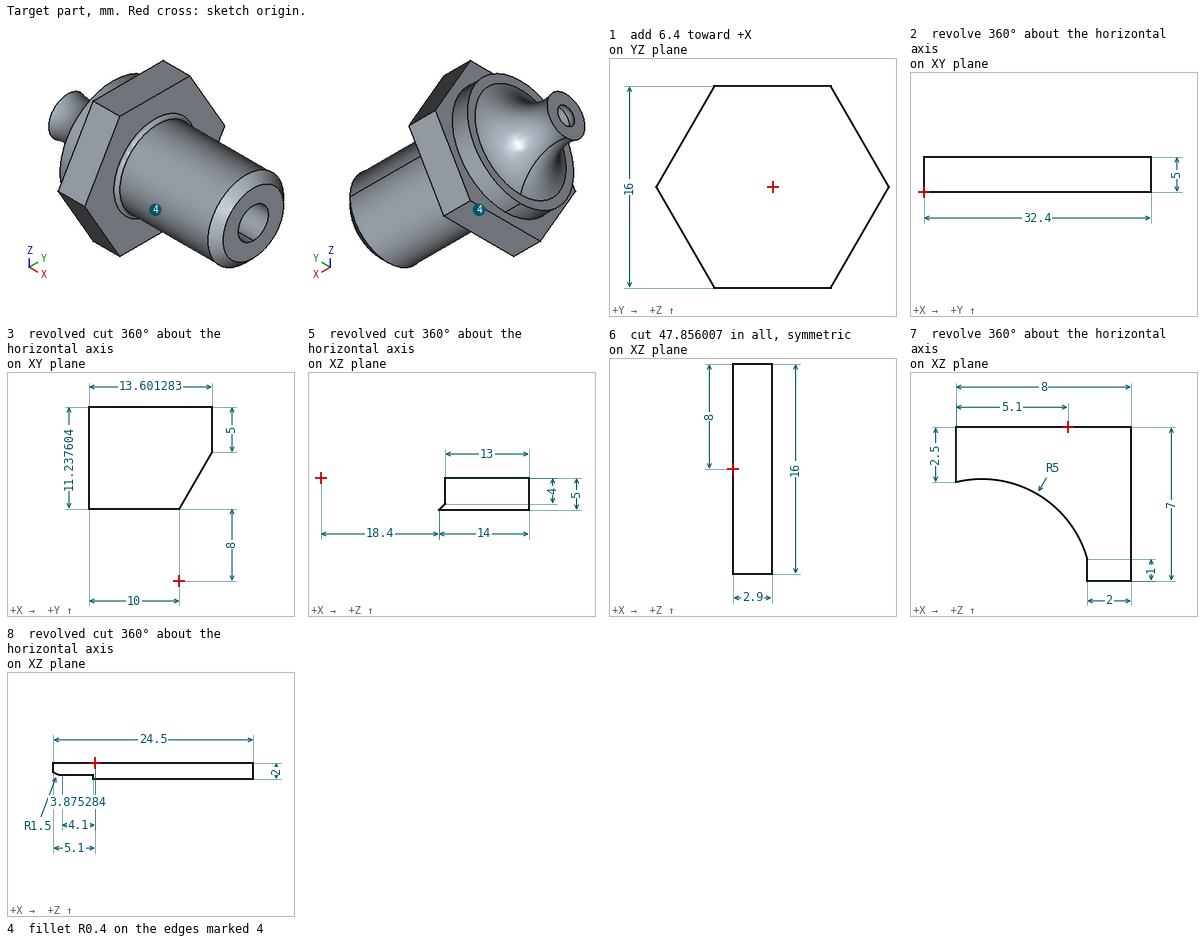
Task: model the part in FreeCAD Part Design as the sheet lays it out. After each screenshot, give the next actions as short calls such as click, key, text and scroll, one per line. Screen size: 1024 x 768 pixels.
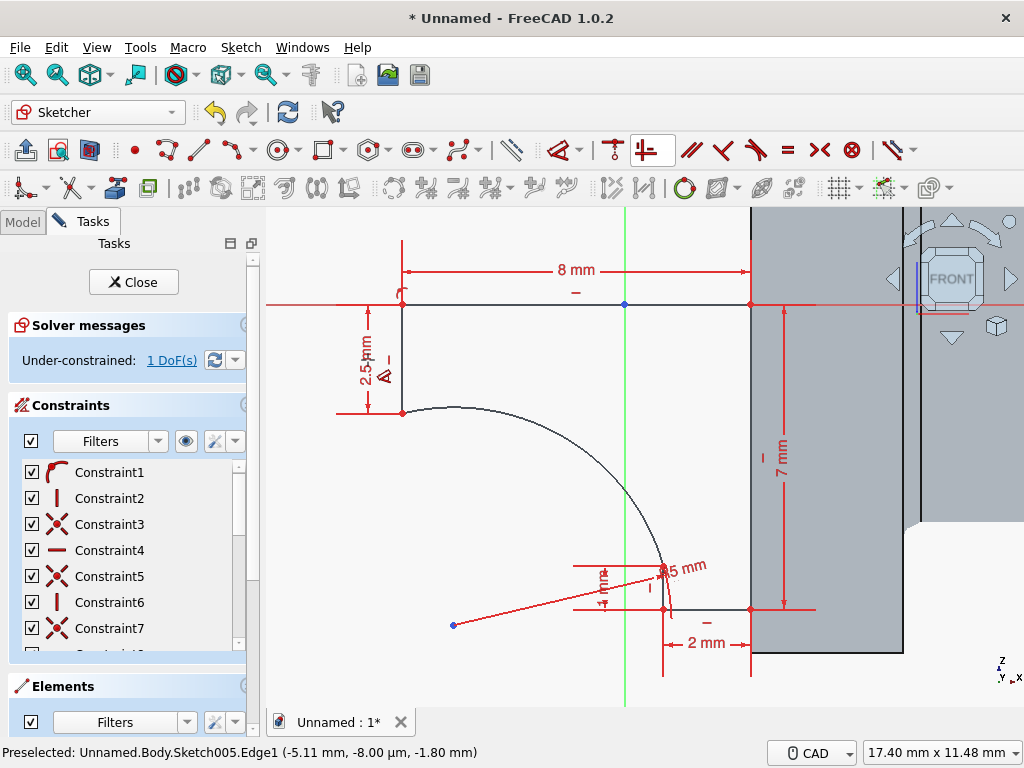
click(402, 414)
click(462, 271)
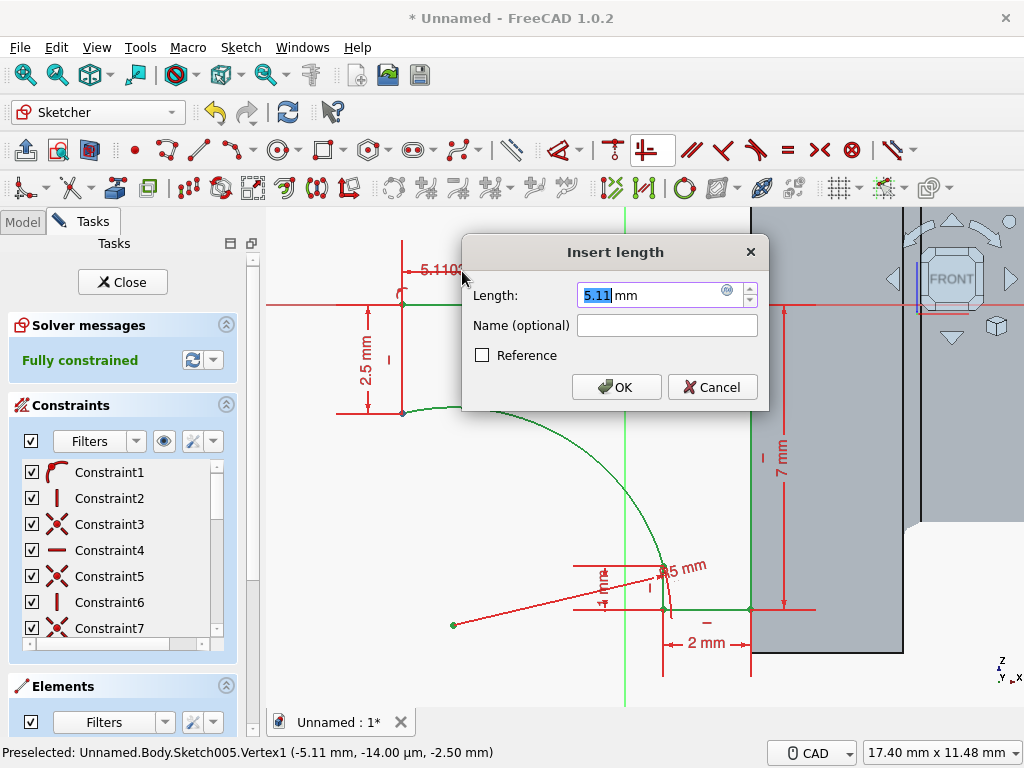
text(5.1)
key(Return)
key(Escape)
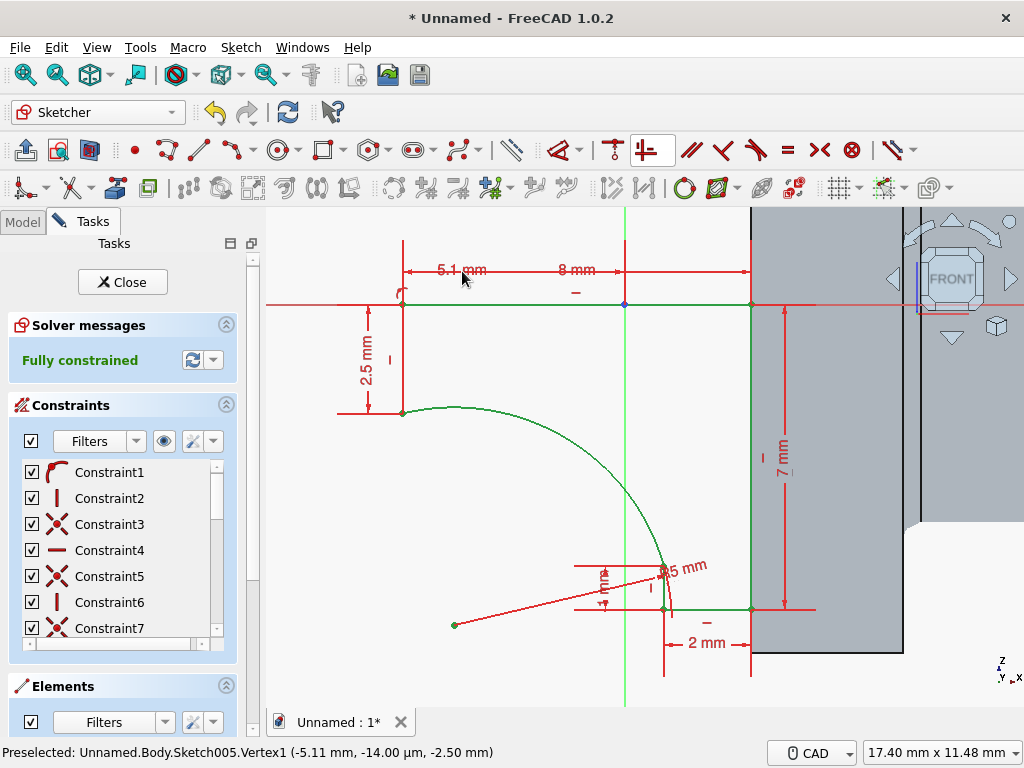
click(123, 282)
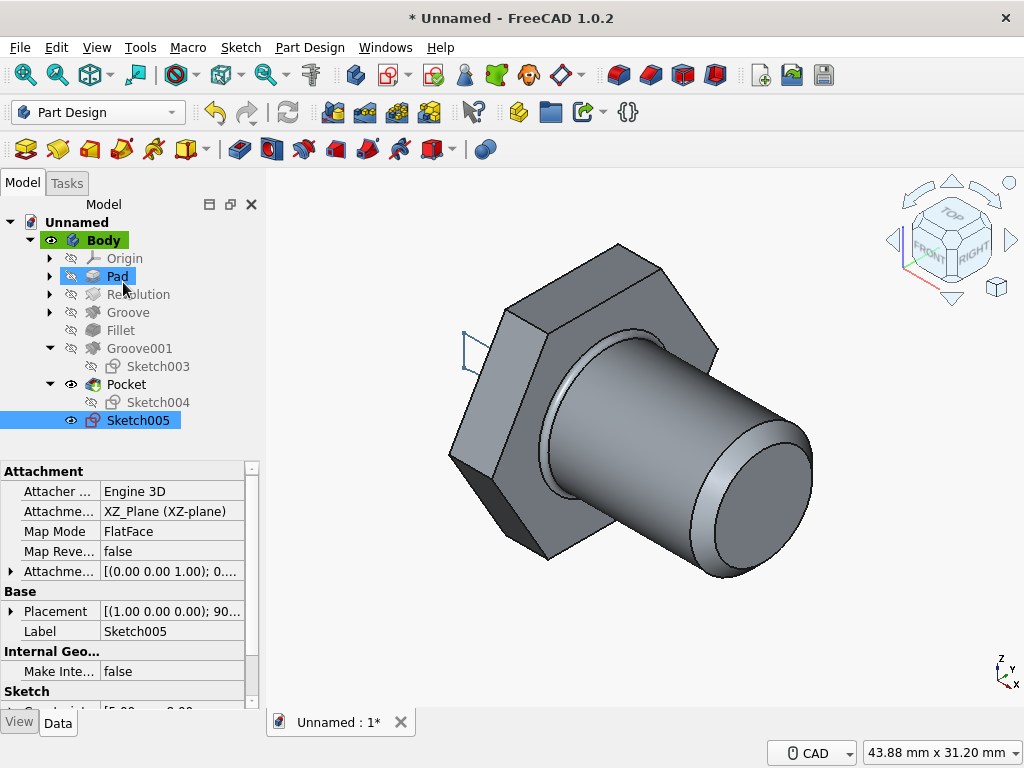
click(58, 150)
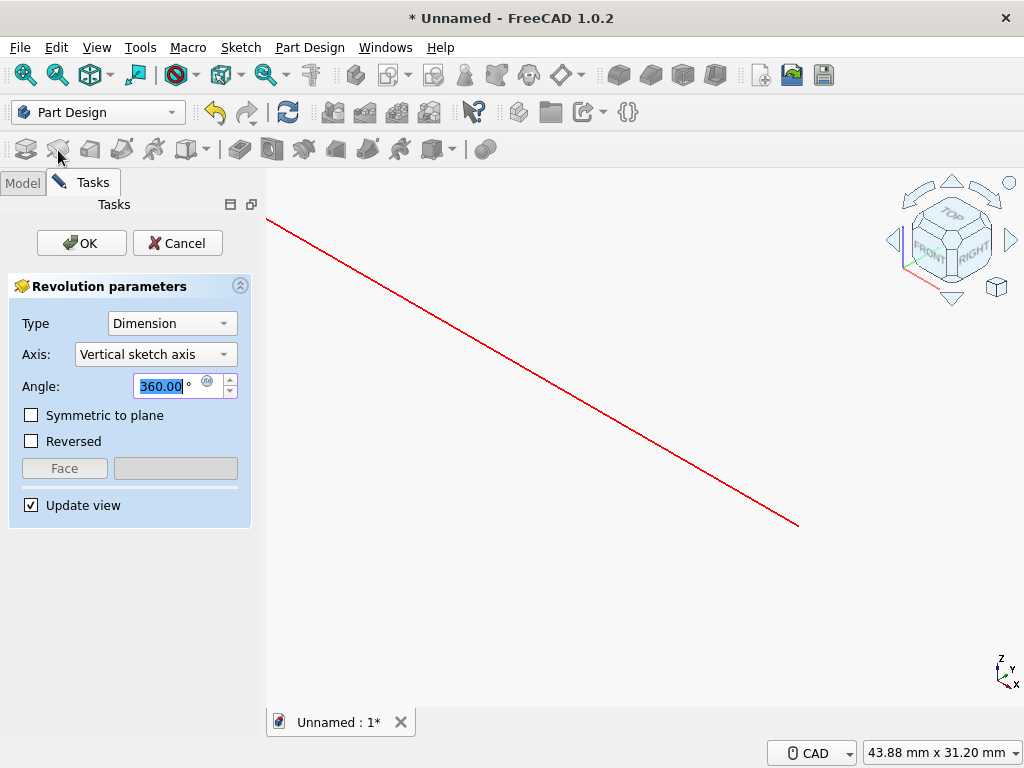
click(156, 354)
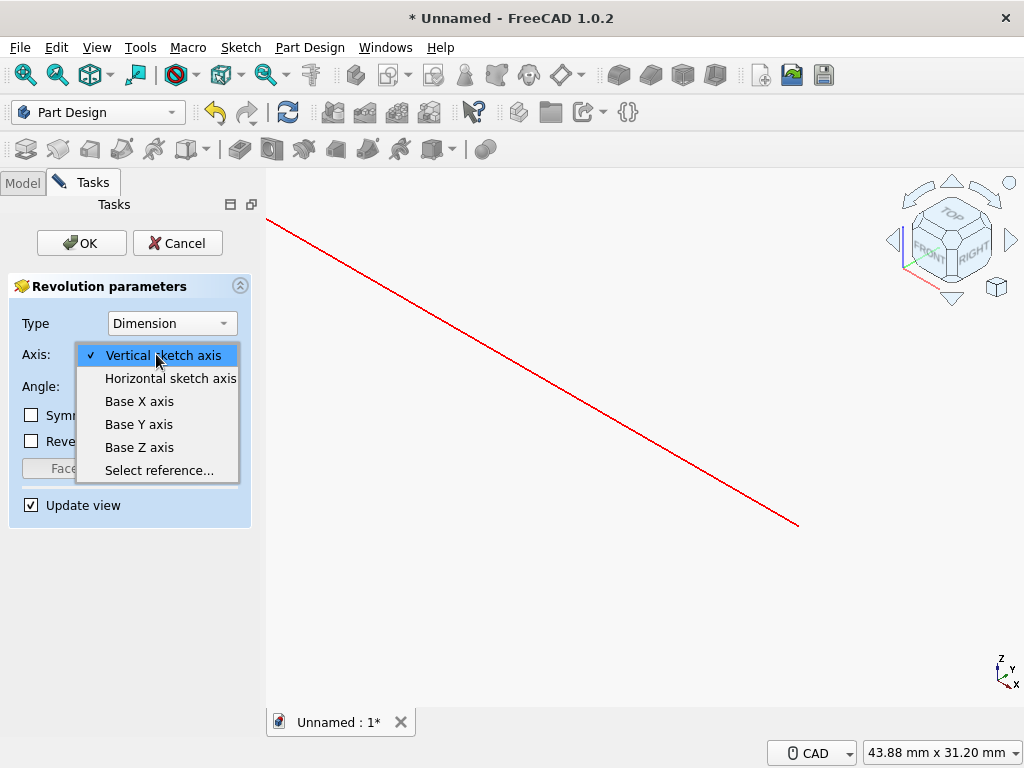
click(156, 378)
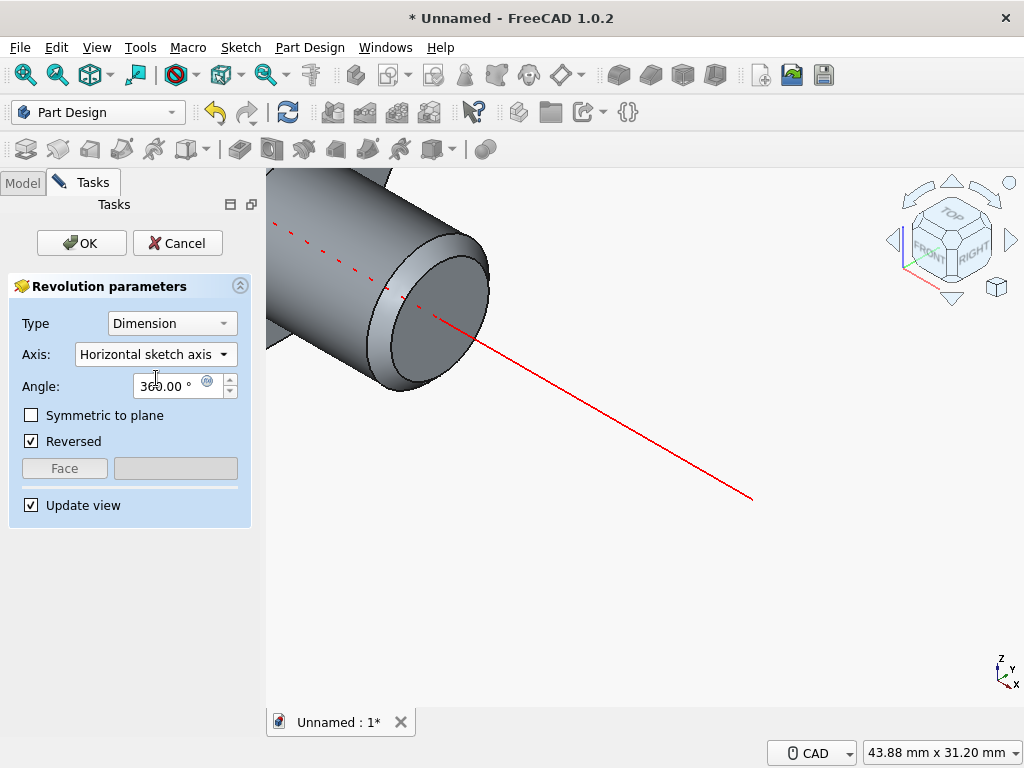
click(82, 243)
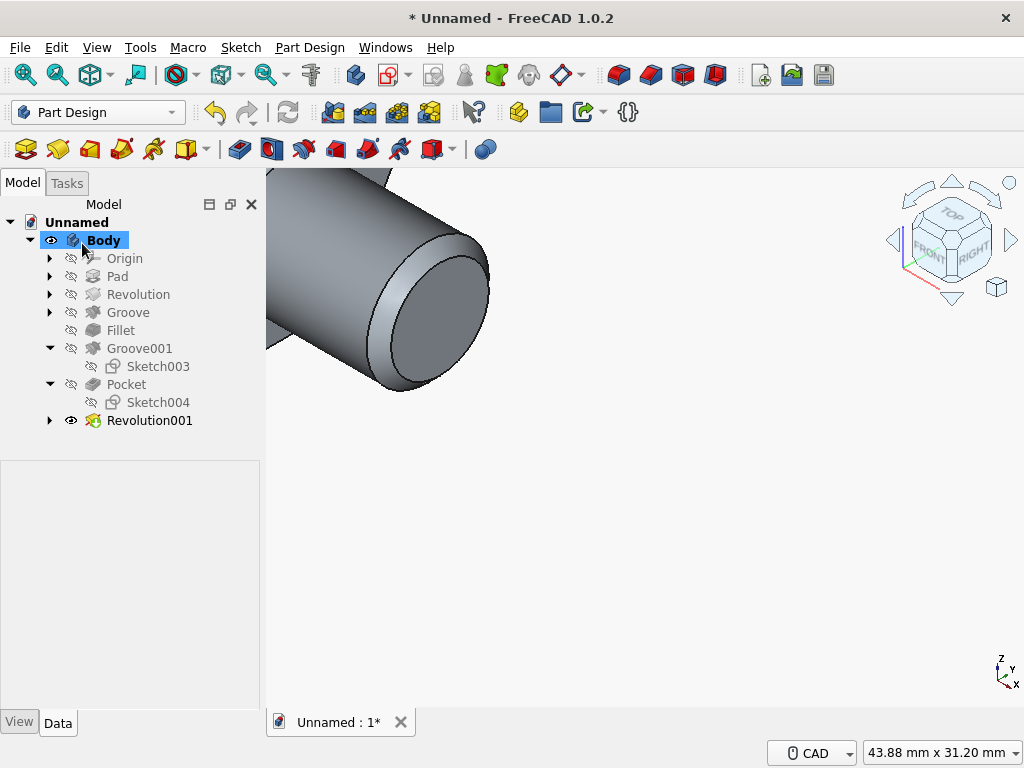
click(26, 76)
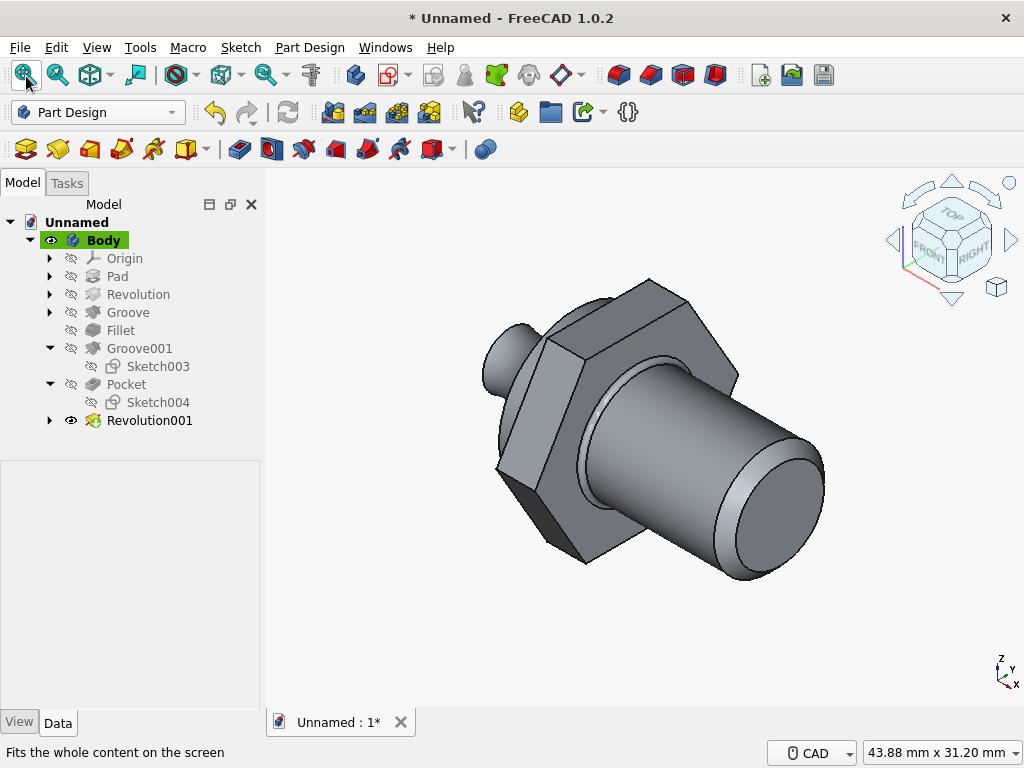
click(388, 76)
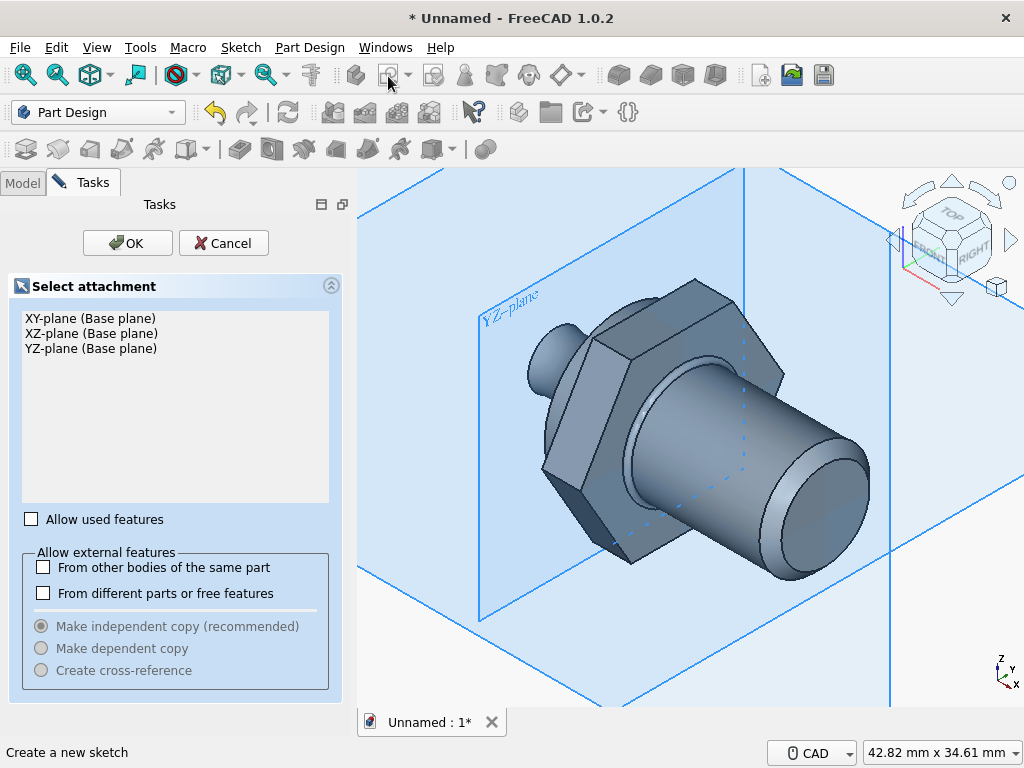
click(82, 334)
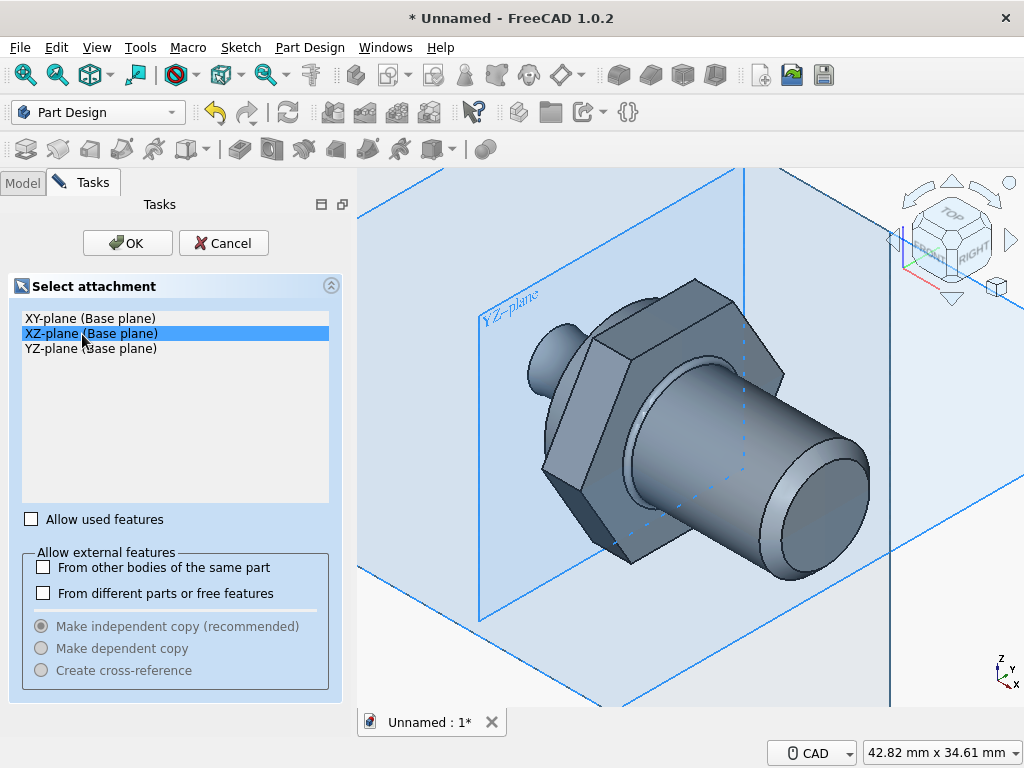
click(128, 243)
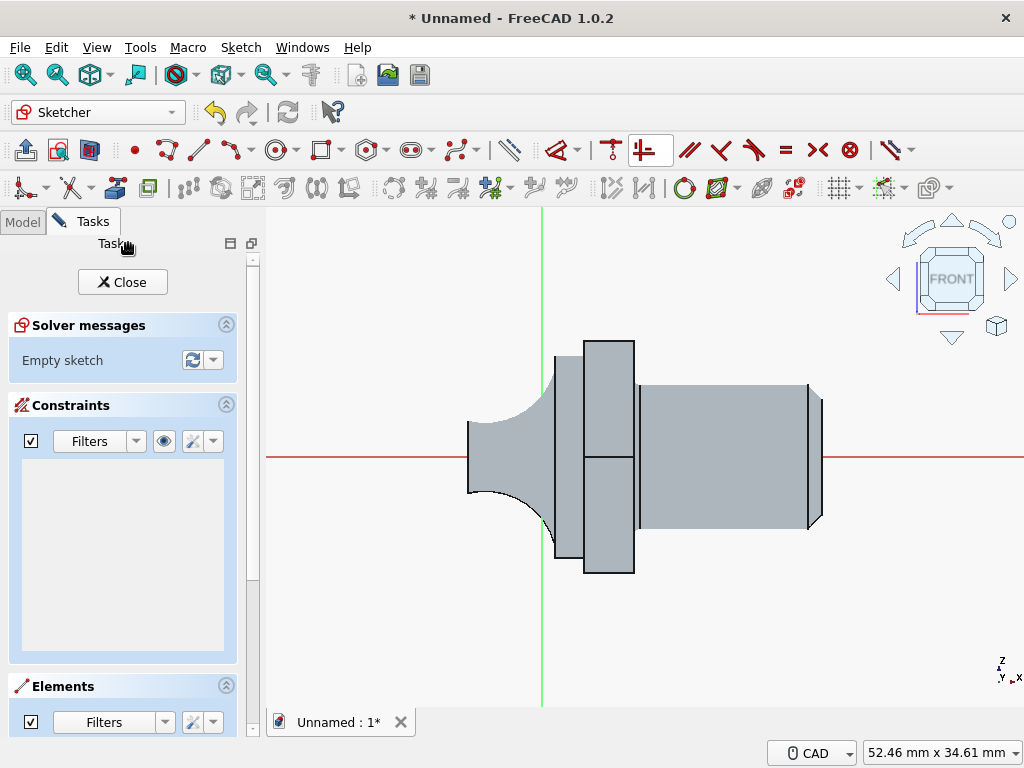
click(90, 150)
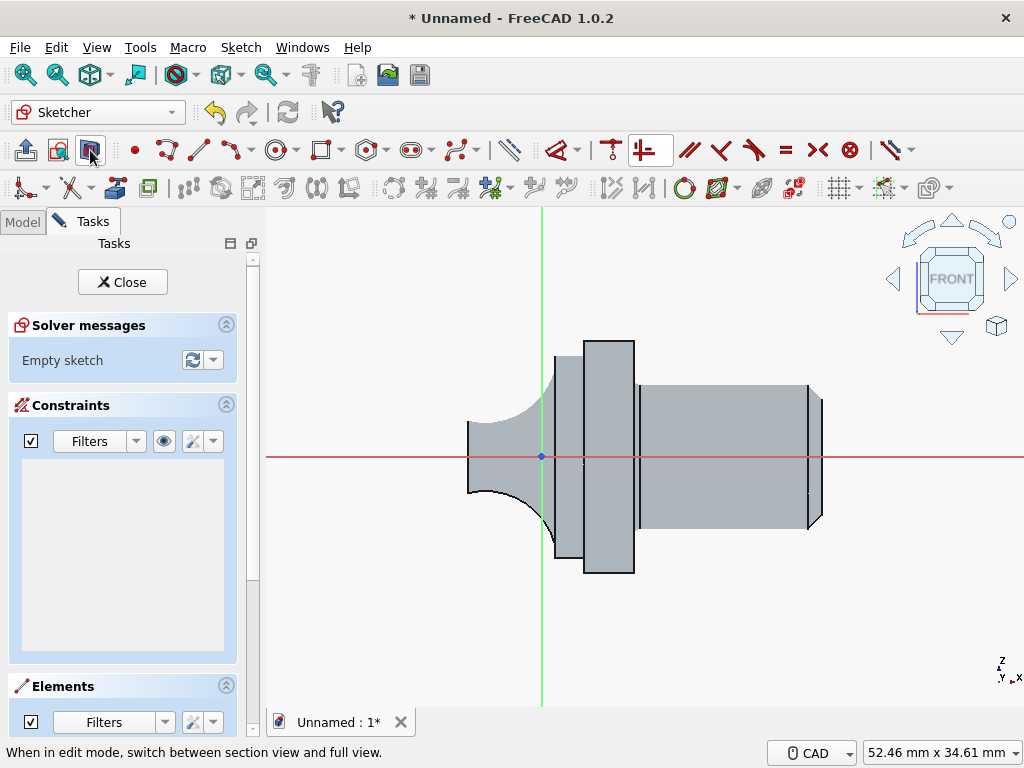
click(168, 150)